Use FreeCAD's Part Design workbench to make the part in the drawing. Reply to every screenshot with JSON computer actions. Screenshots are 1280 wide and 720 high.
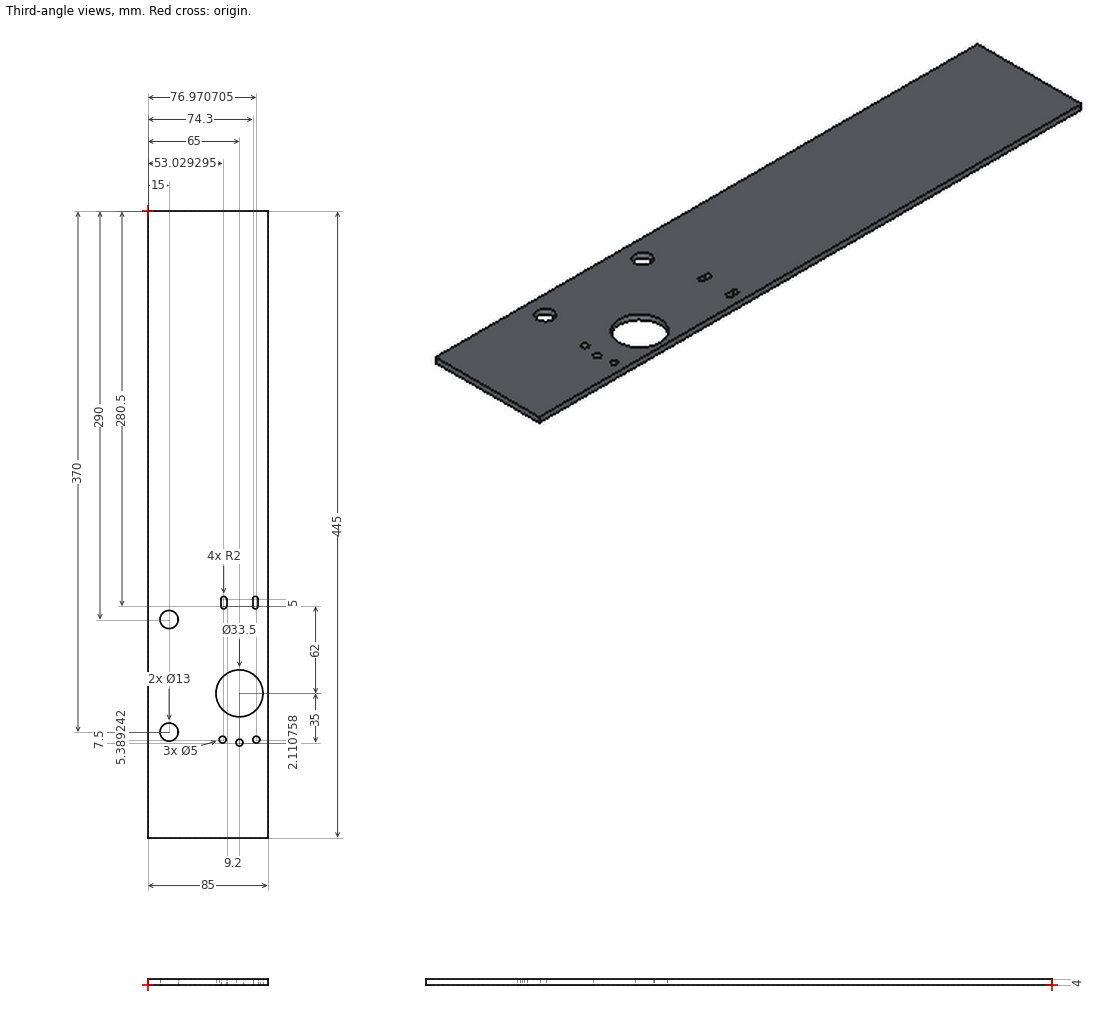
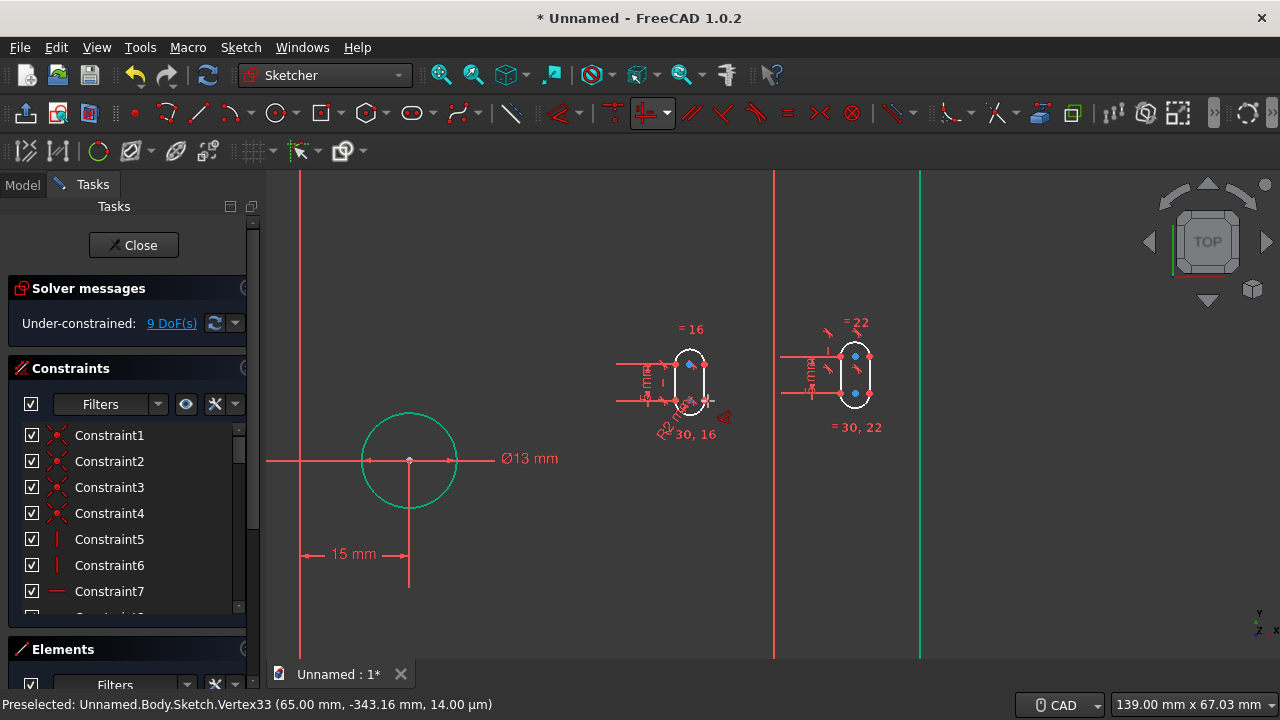
{"action": "left_click", "coordinate": [704, 401]}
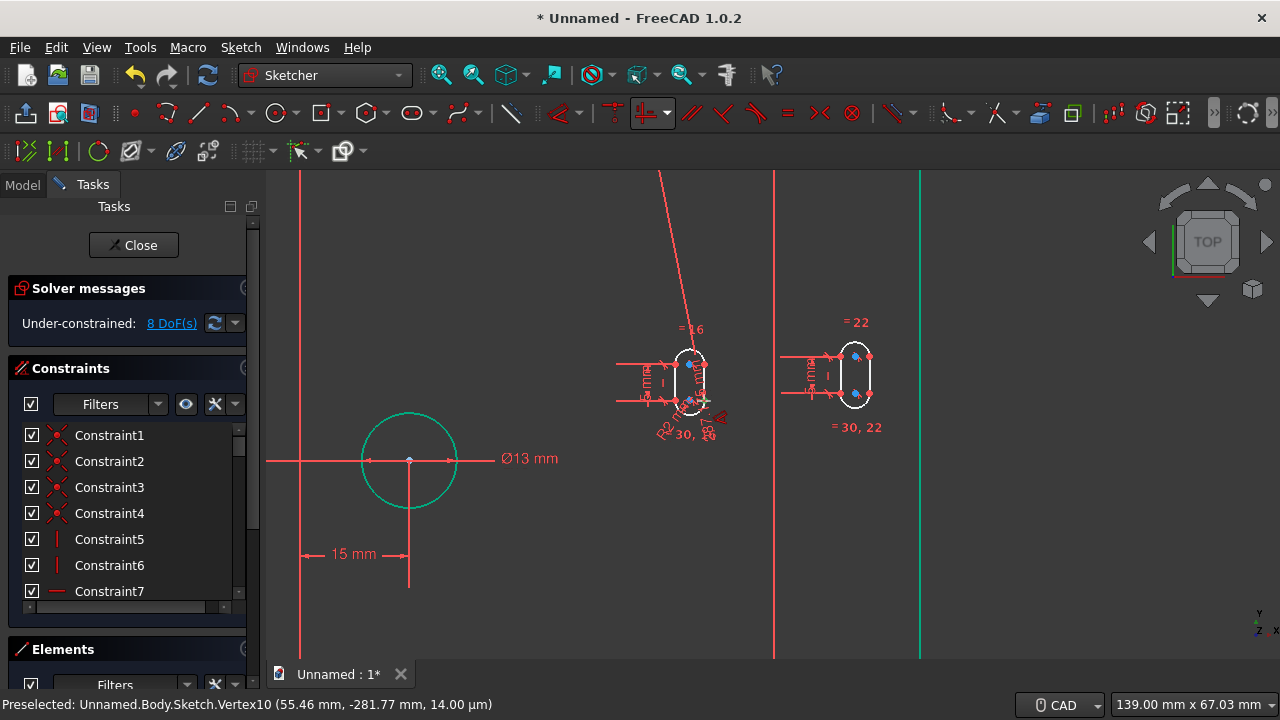
{"action": "scroll", "coordinate": [714, 459], "scroll_direction": "down", "scroll_amount": 12}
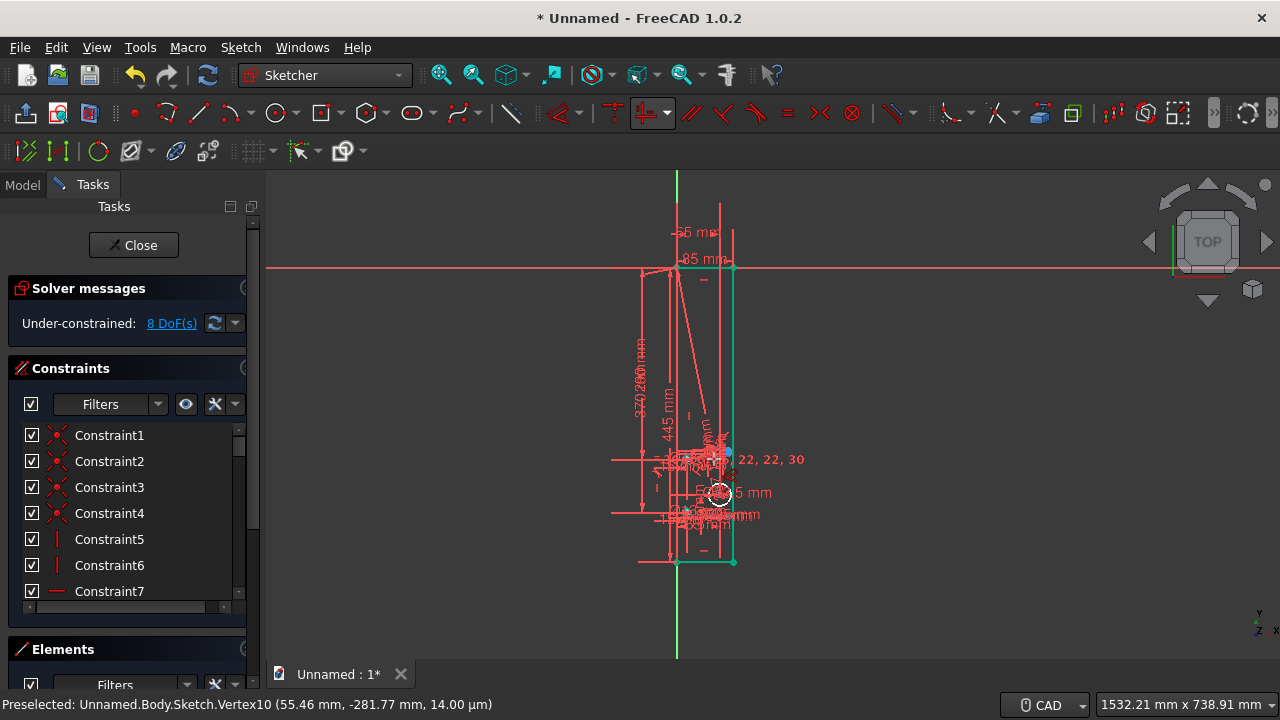
{"action": "left_click", "coordinate": [720, 495]}
{"action": "left_click", "coordinate": [754, 484]}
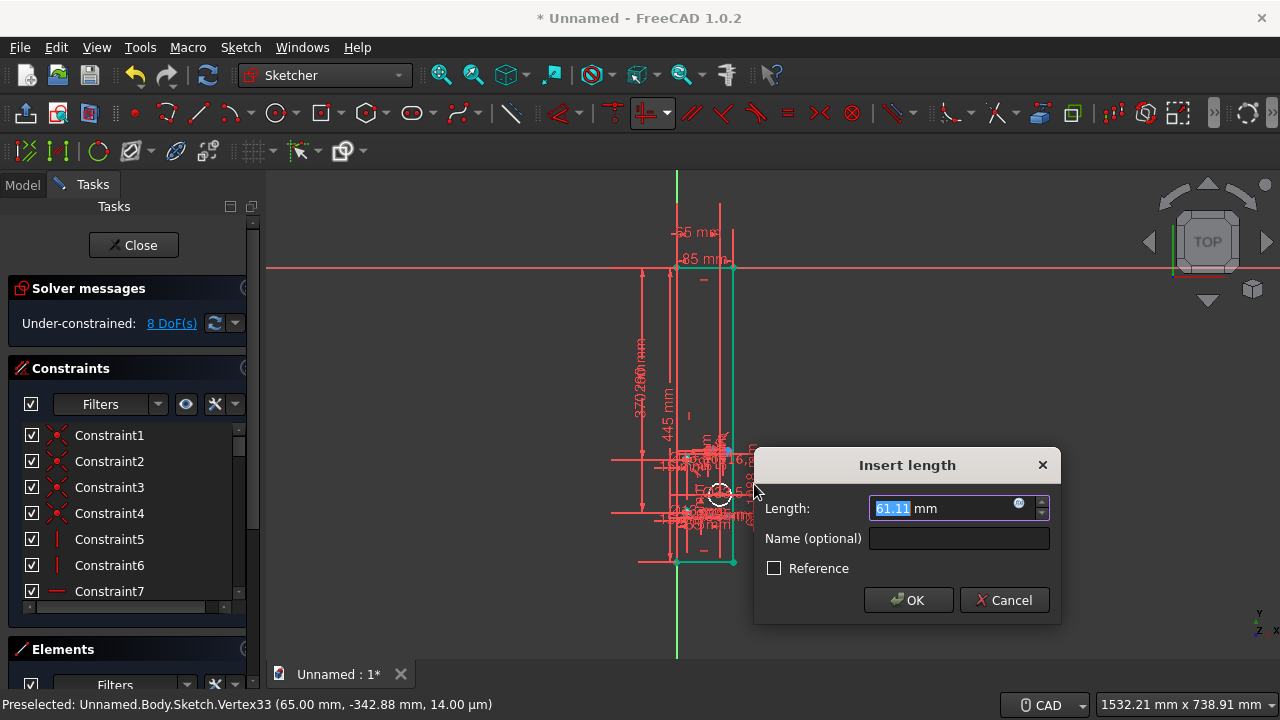
{"action": "type", "text": "62"}
{"action": "key", "text": "Return"}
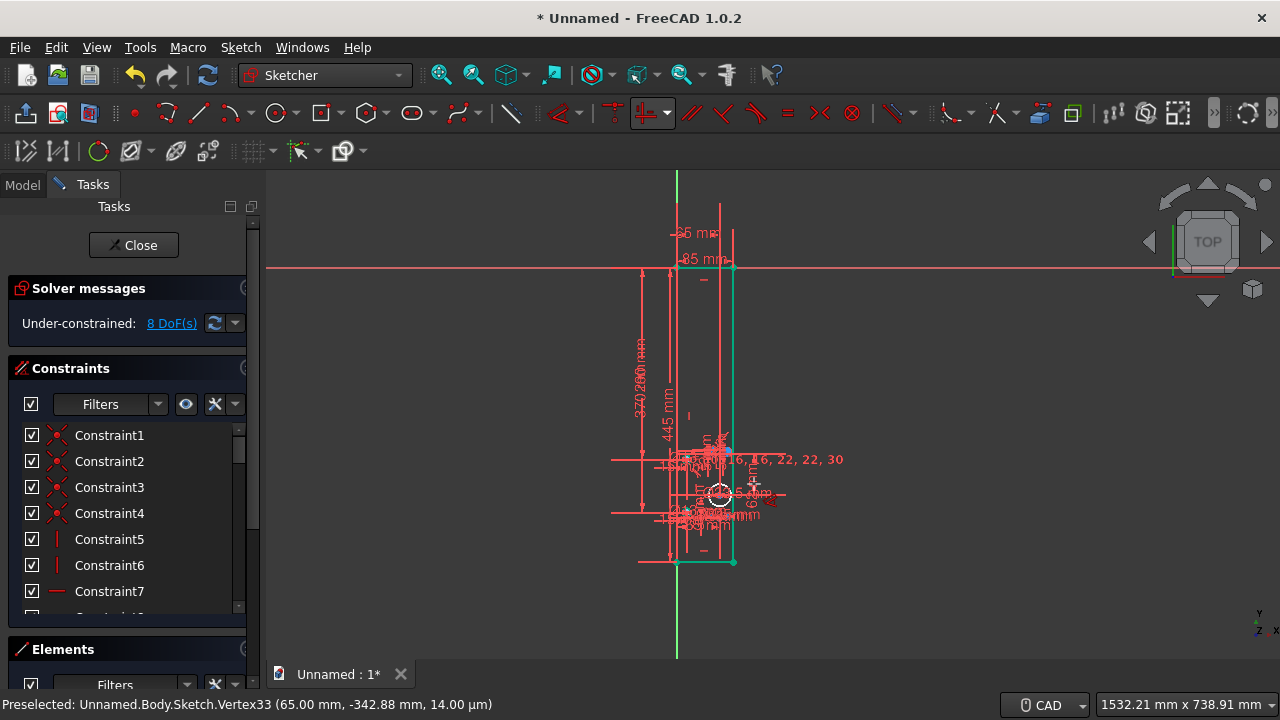
{"action": "scroll", "coordinate": [687, 513], "scroll_direction": "up", "scroll_amount": 11}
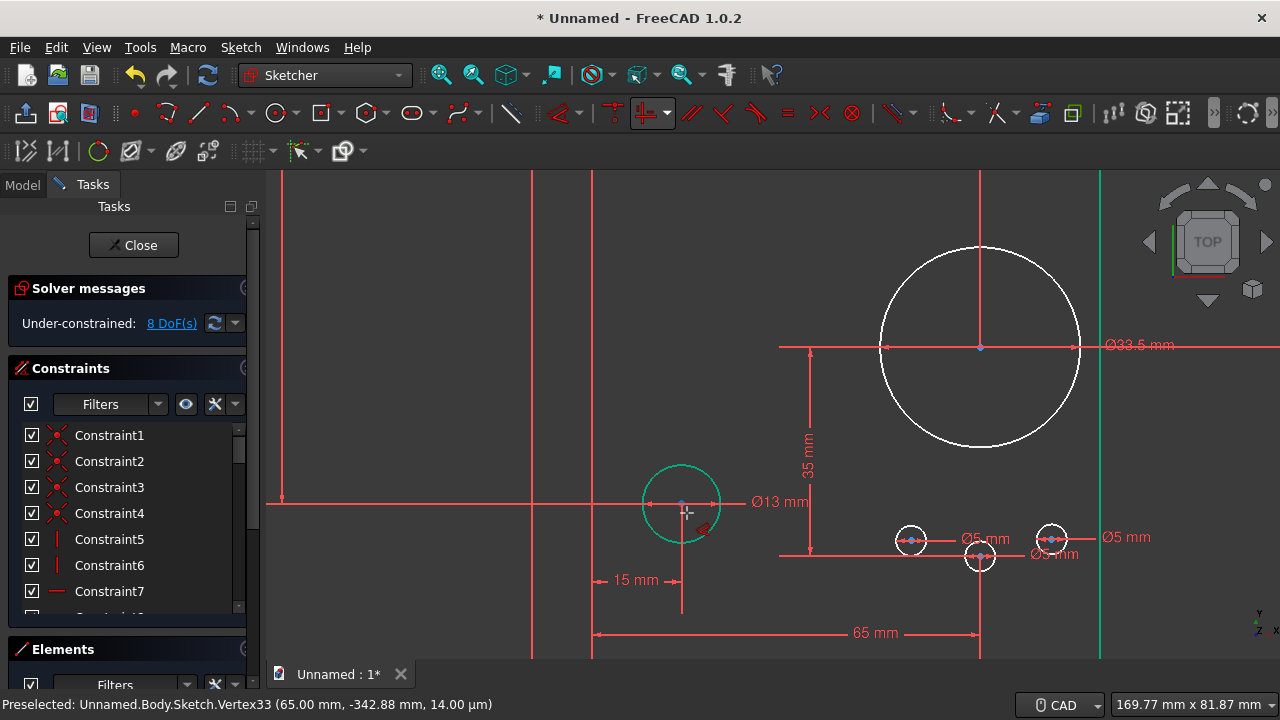
{"action": "left_click", "coordinate": [682, 504]}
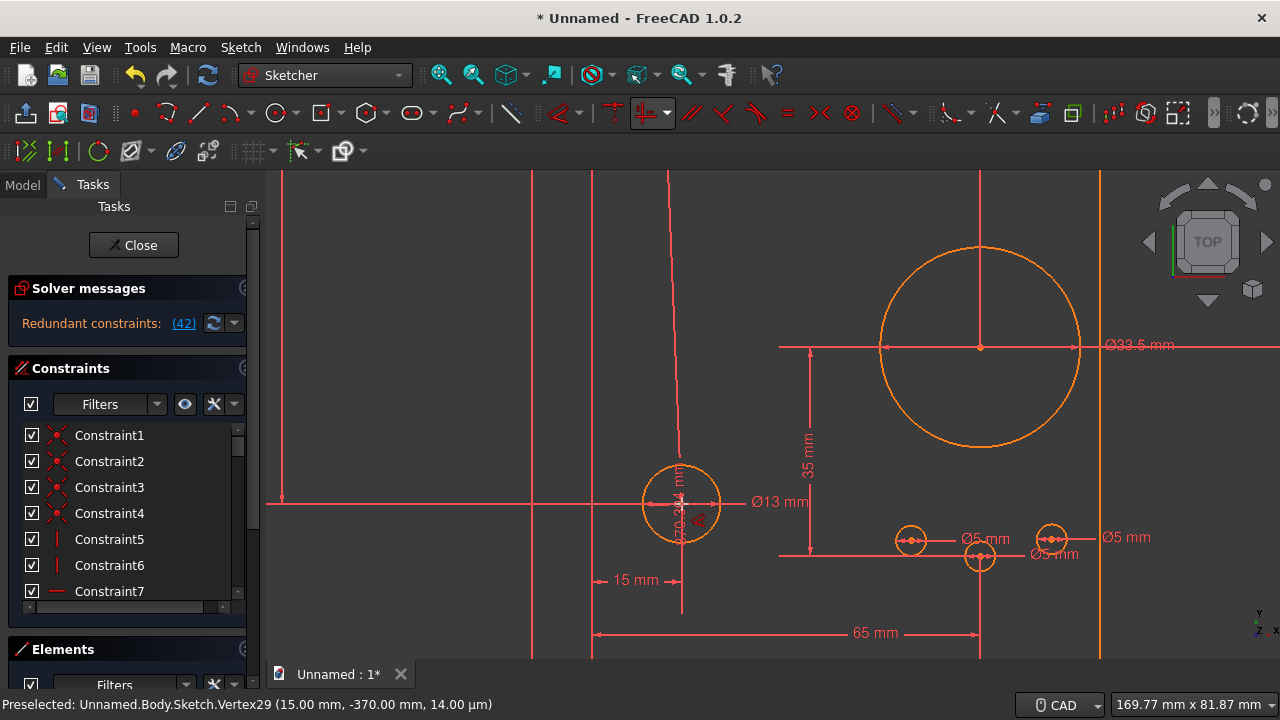
{"action": "left_click", "coordinate": [980, 556]}
{"action": "left_click", "coordinate": [648, 548]}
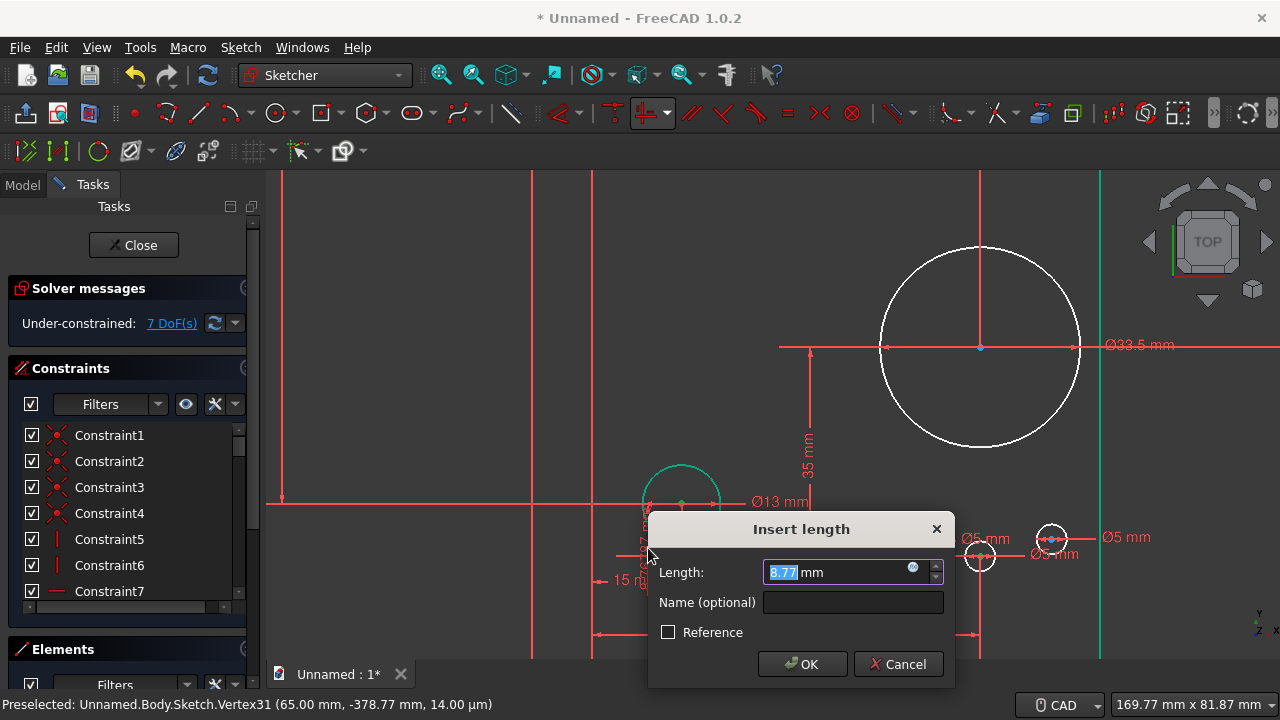
{"action": "type", "text": "7.5"}
{"action": "key", "text": "Return"}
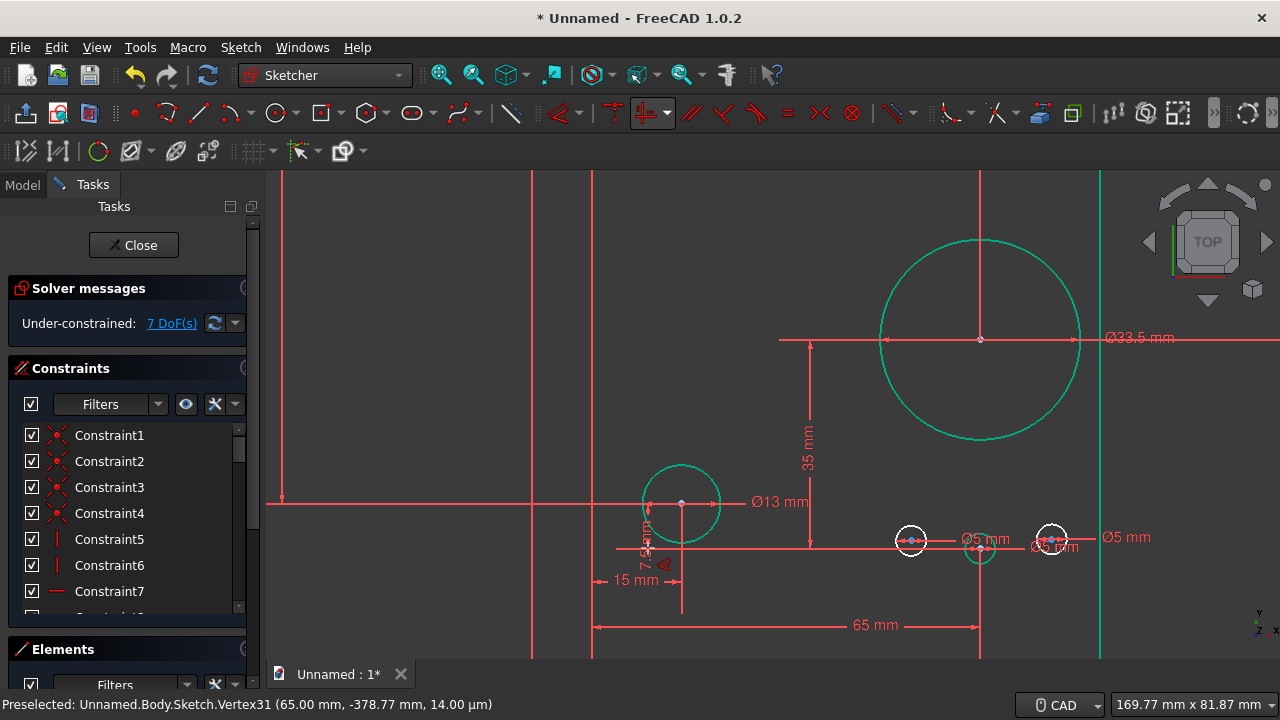
{"action": "scroll", "coordinate": [687, 513], "scroll_direction": "down", "scroll_amount": 11}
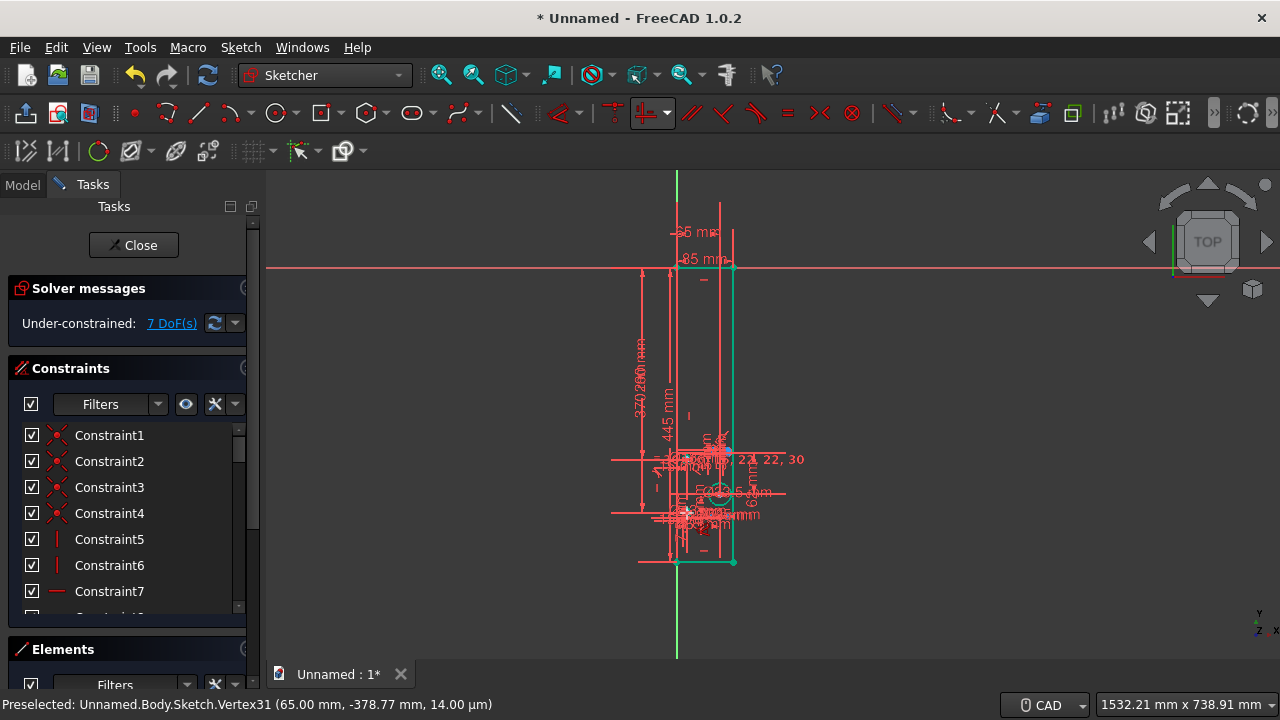
{"action": "scroll", "coordinate": [714, 453], "scroll_direction": "up", "scroll_amount": 12}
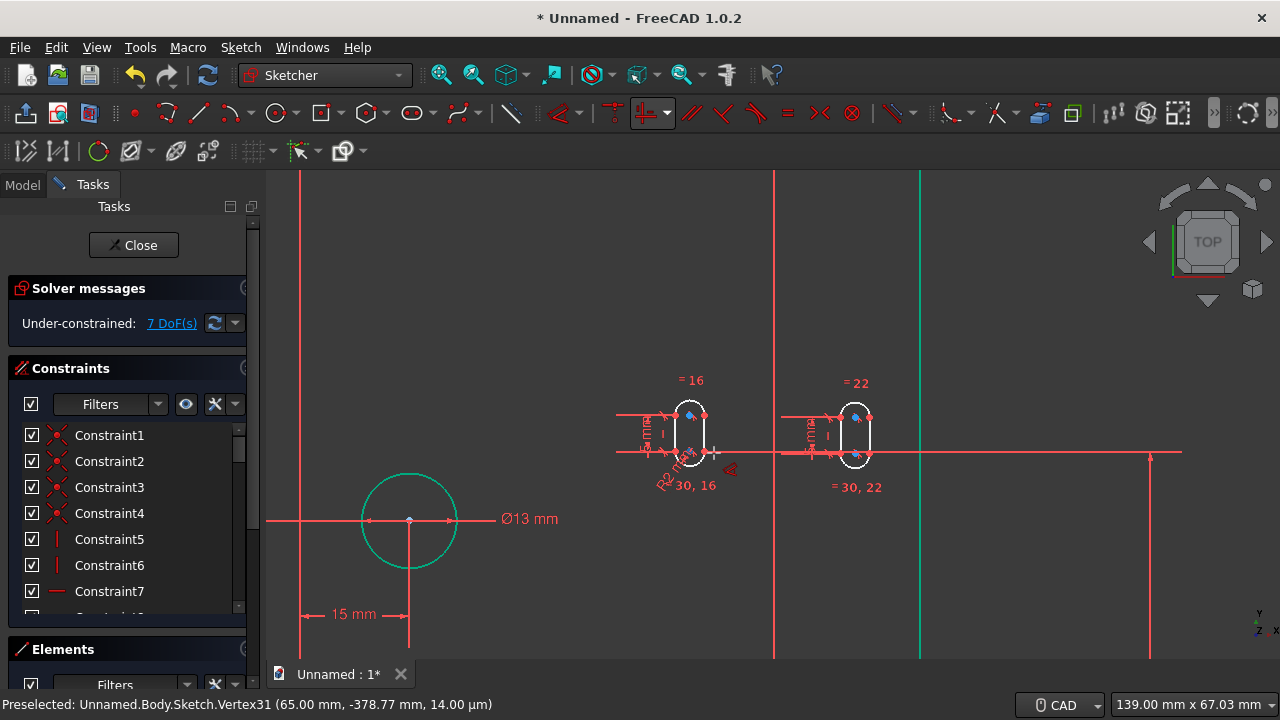
{"action": "left_click", "coordinate": [704, 452]}